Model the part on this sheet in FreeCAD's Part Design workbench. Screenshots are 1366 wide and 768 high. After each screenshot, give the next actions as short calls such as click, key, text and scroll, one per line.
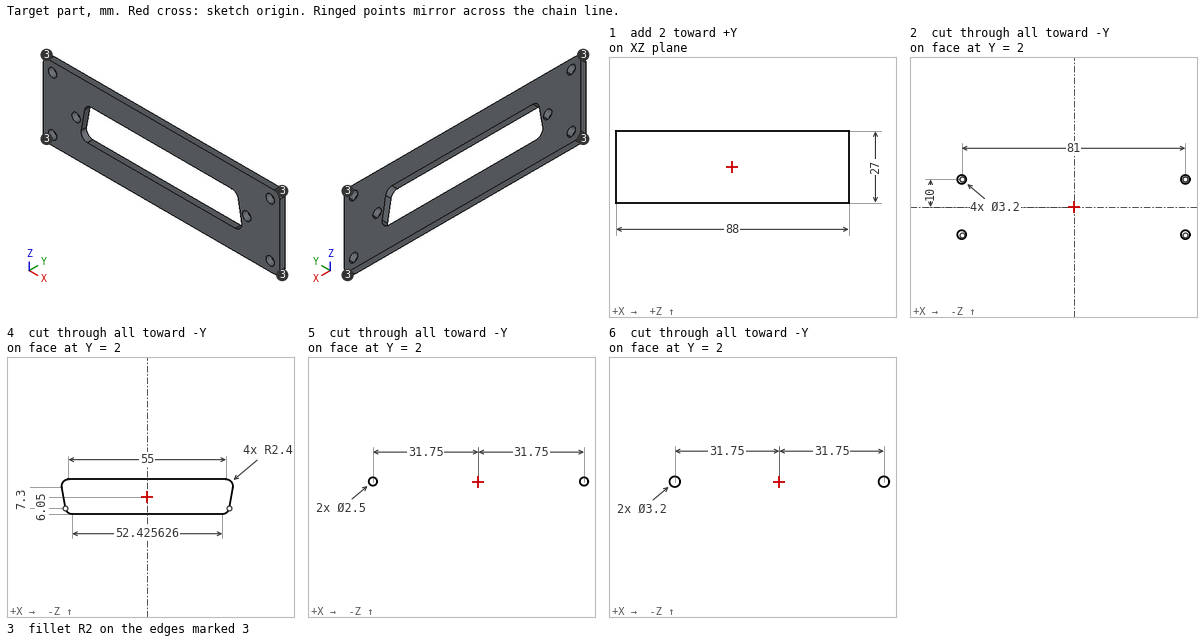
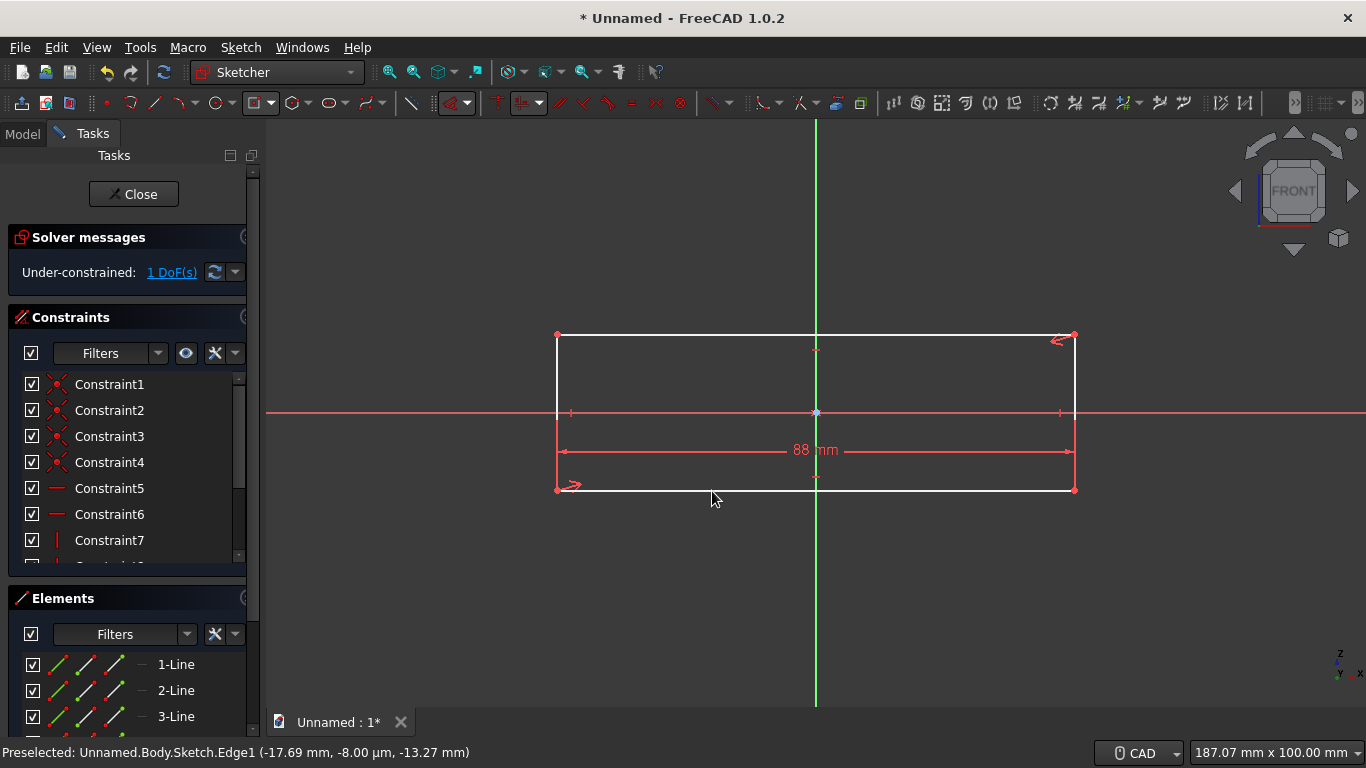
click(1075, 444)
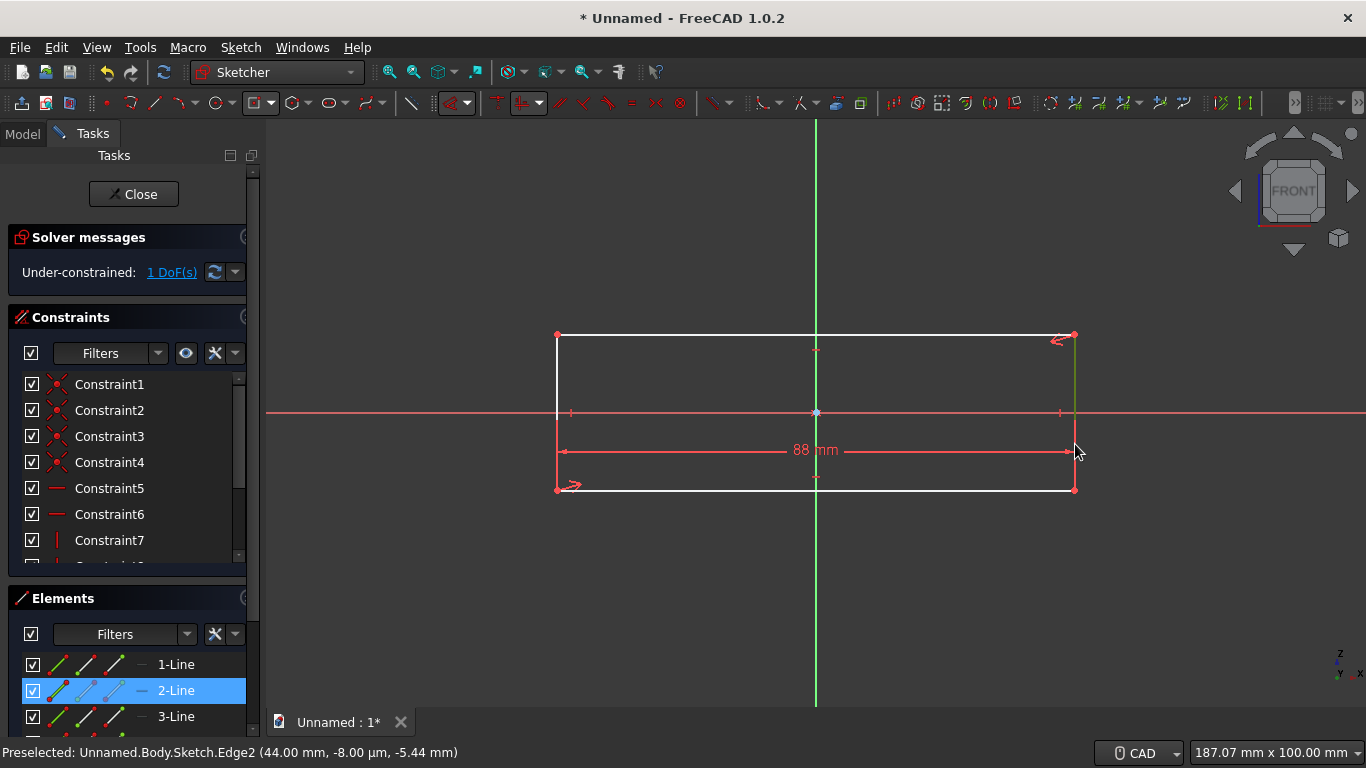
click(470, 104)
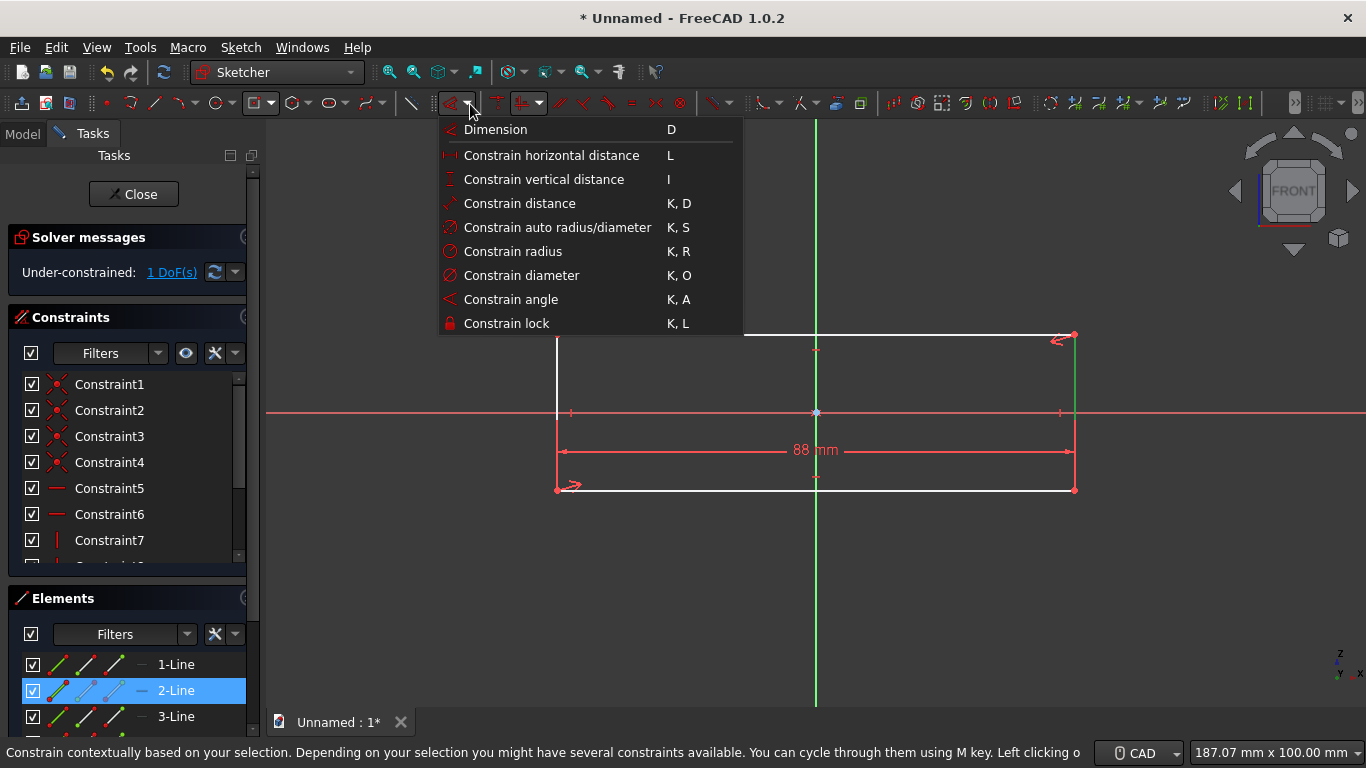
click(591, 179)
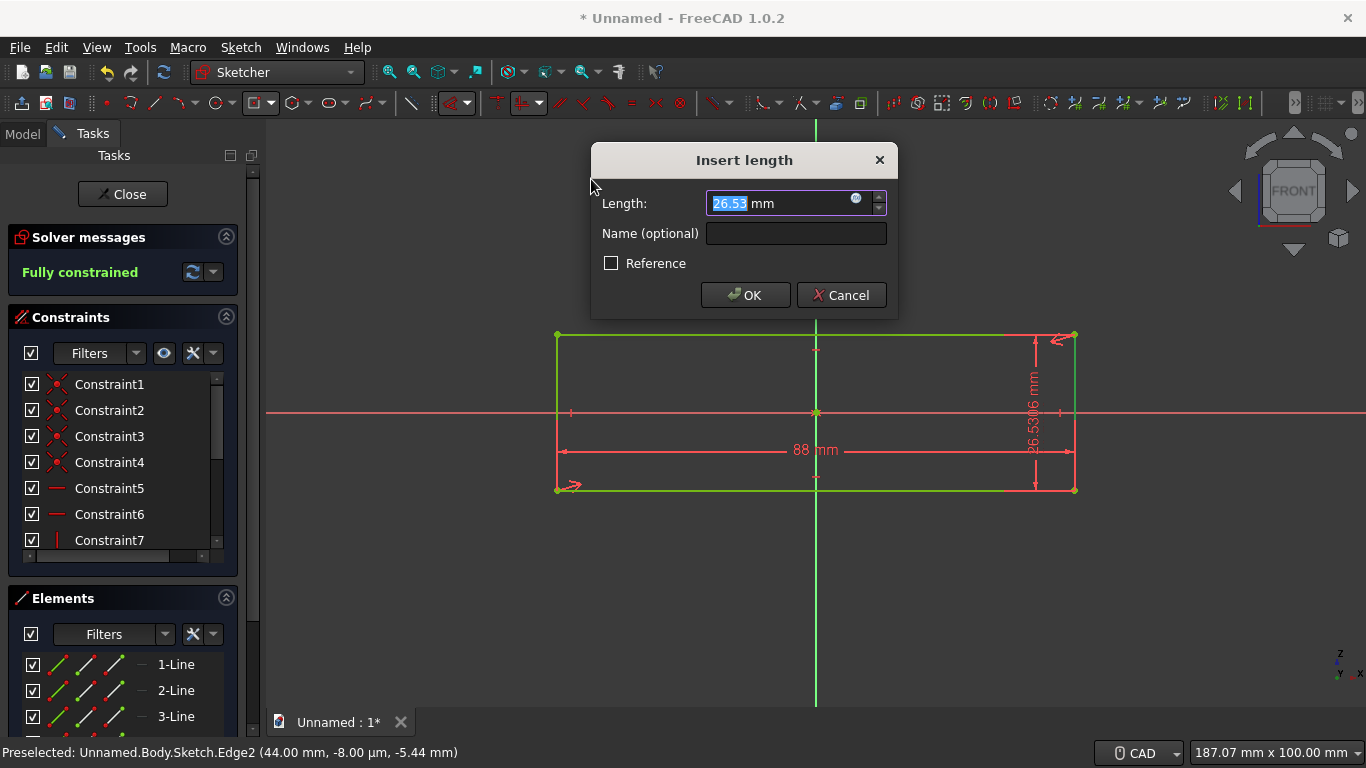
text(27)
key(Return)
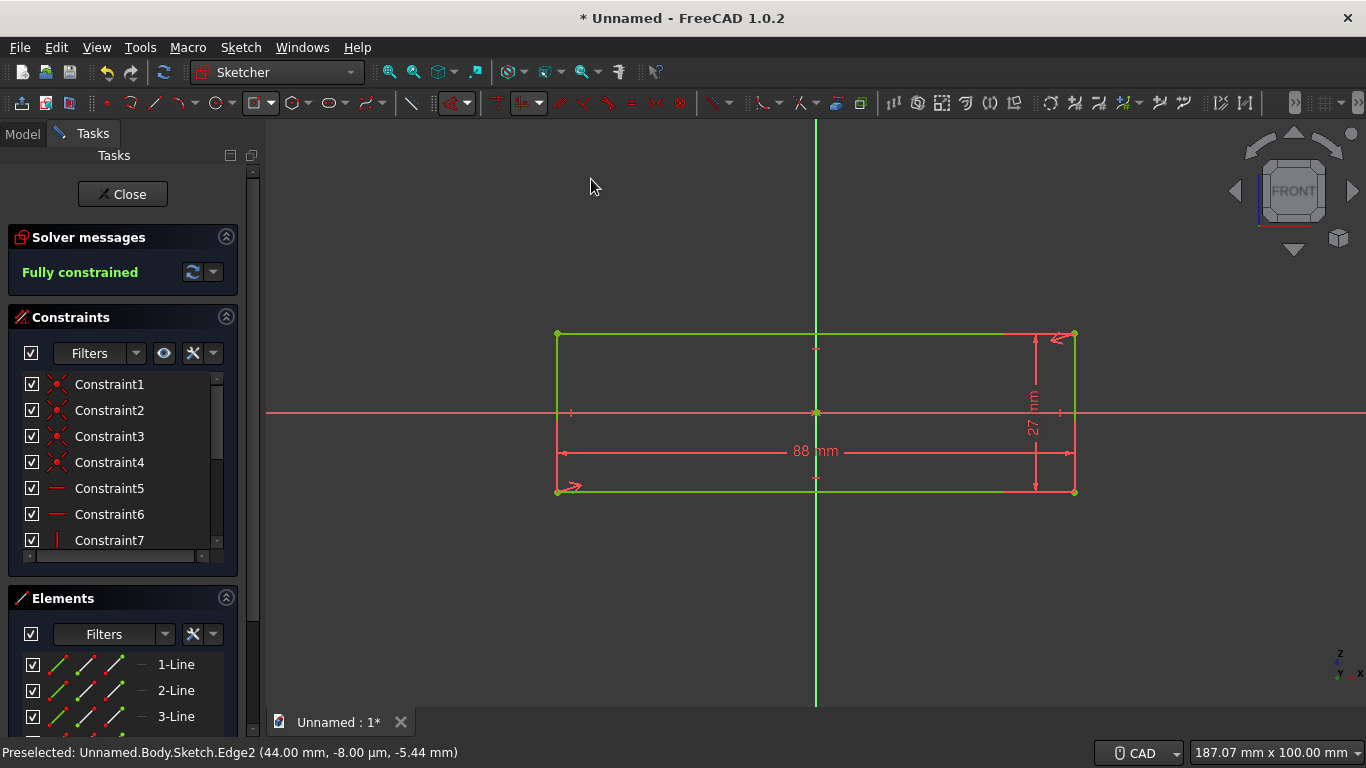
click(123, 194)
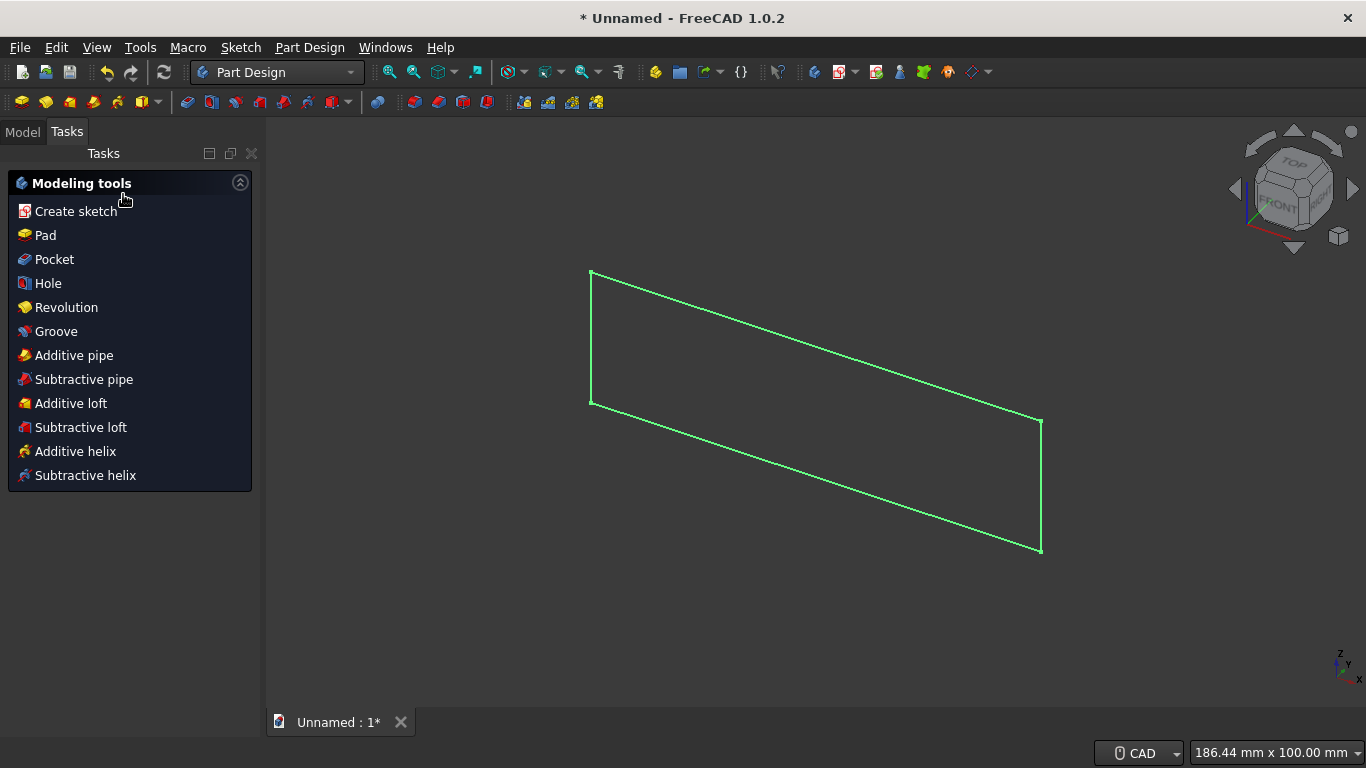
click(22, 102)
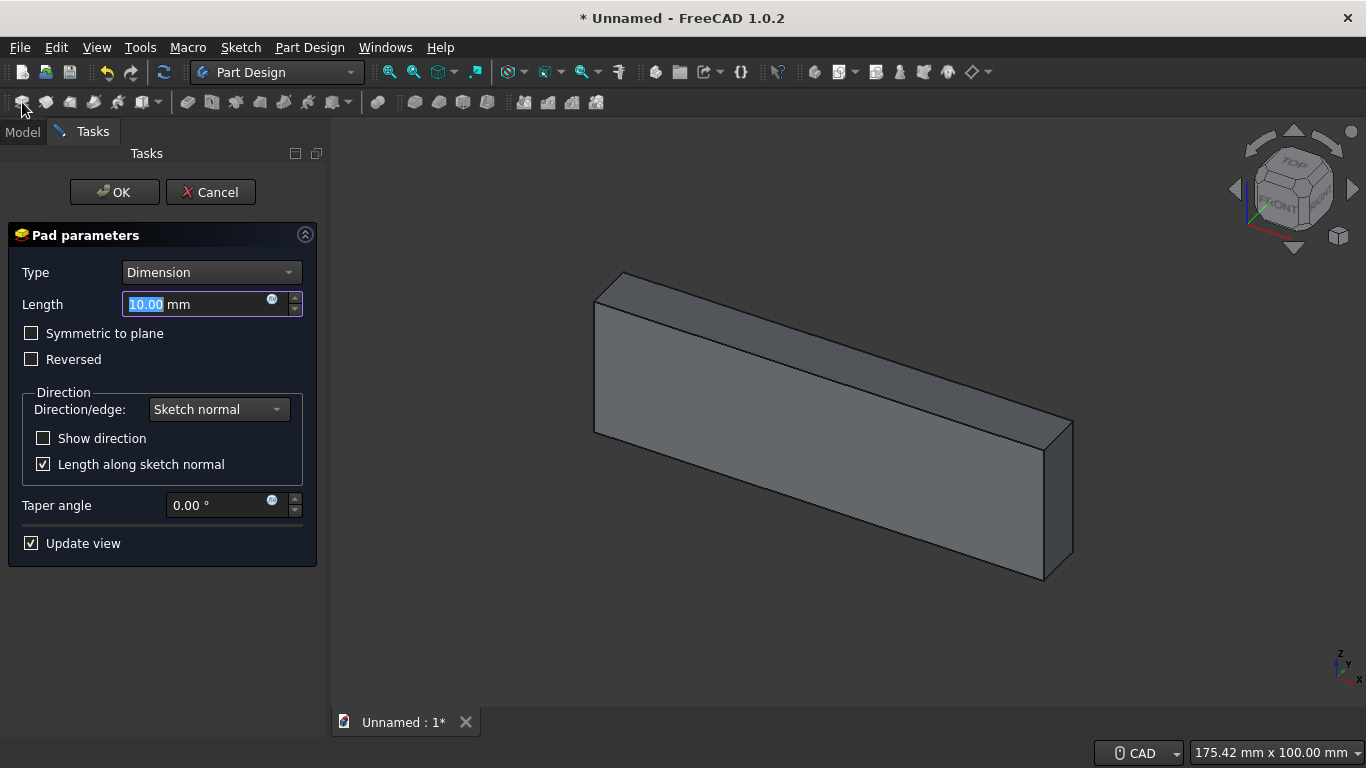
text(2)
key(Tab)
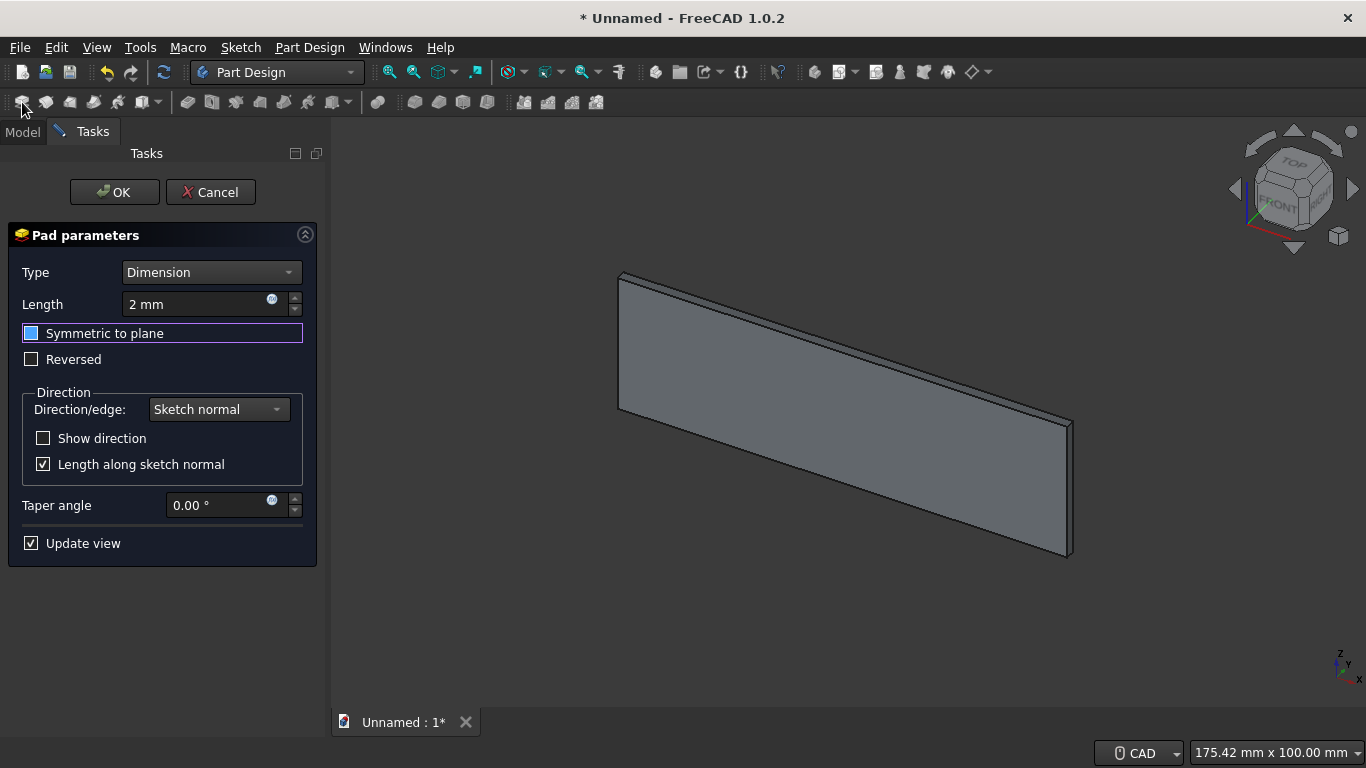
click(30, 359)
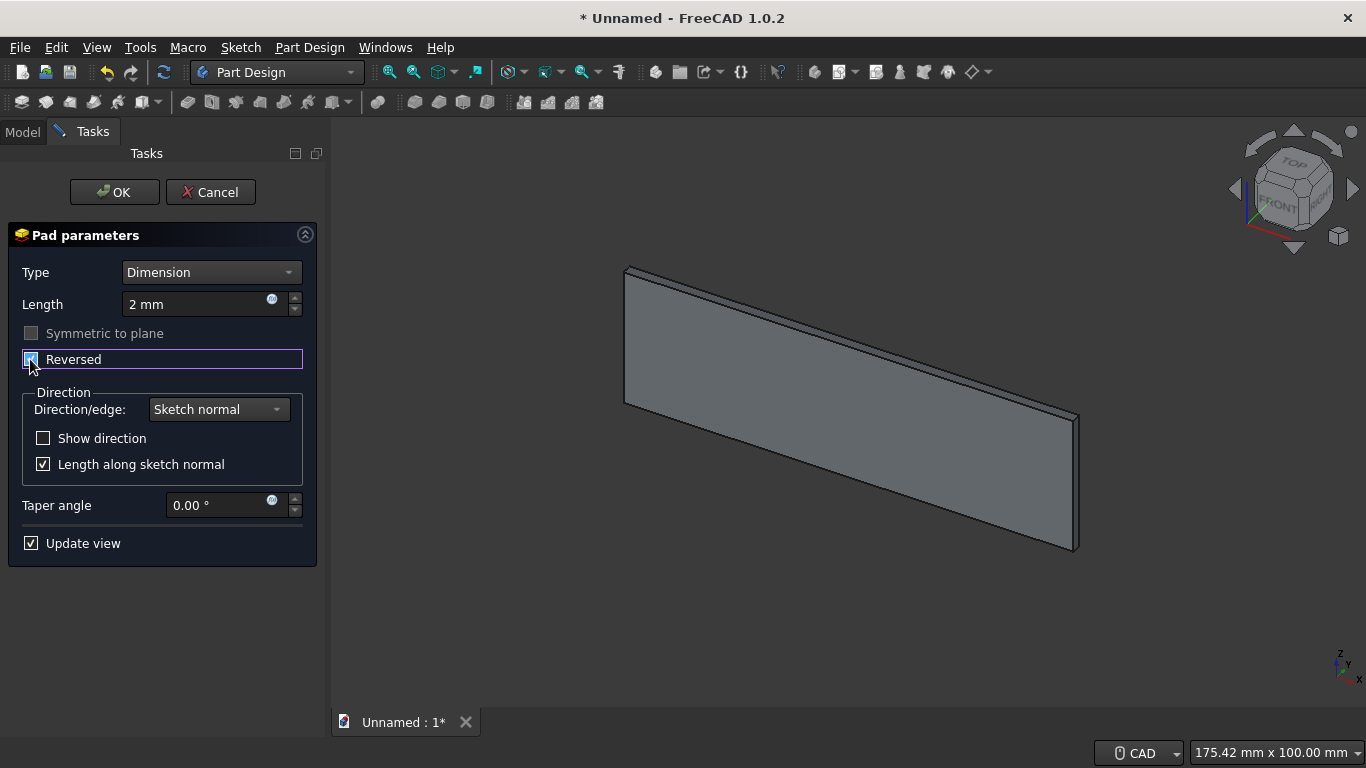
click(115, 192)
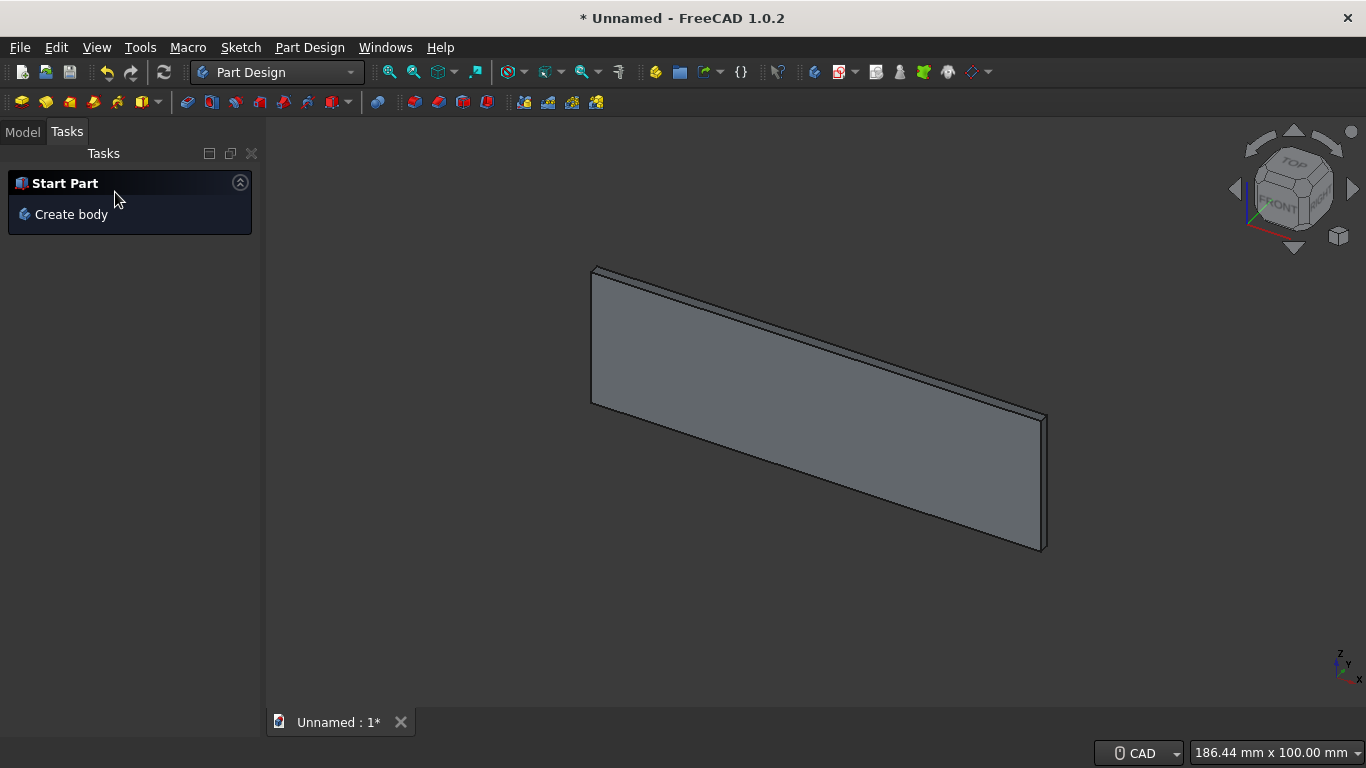
key(4)